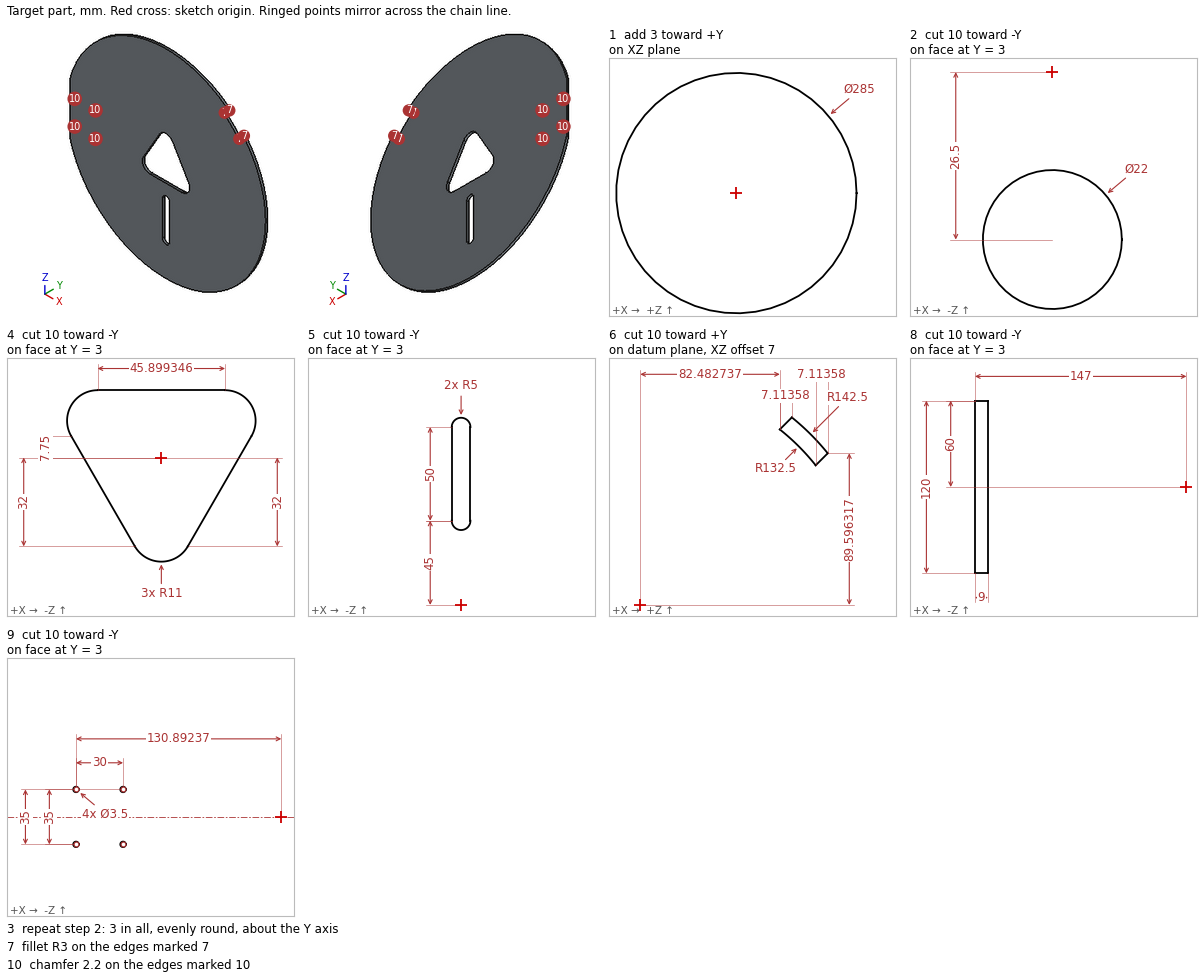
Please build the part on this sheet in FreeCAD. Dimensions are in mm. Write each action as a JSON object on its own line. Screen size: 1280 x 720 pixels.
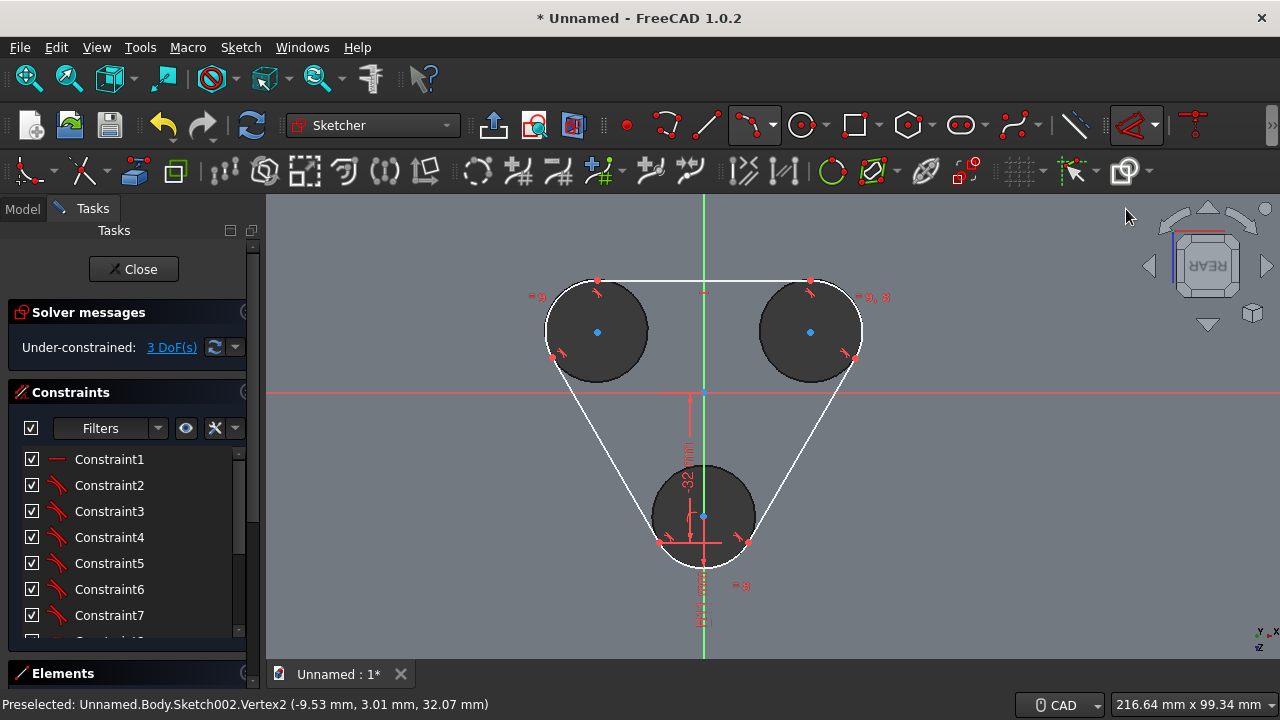
{"action": "left_click", "coordinate": [748, 543]}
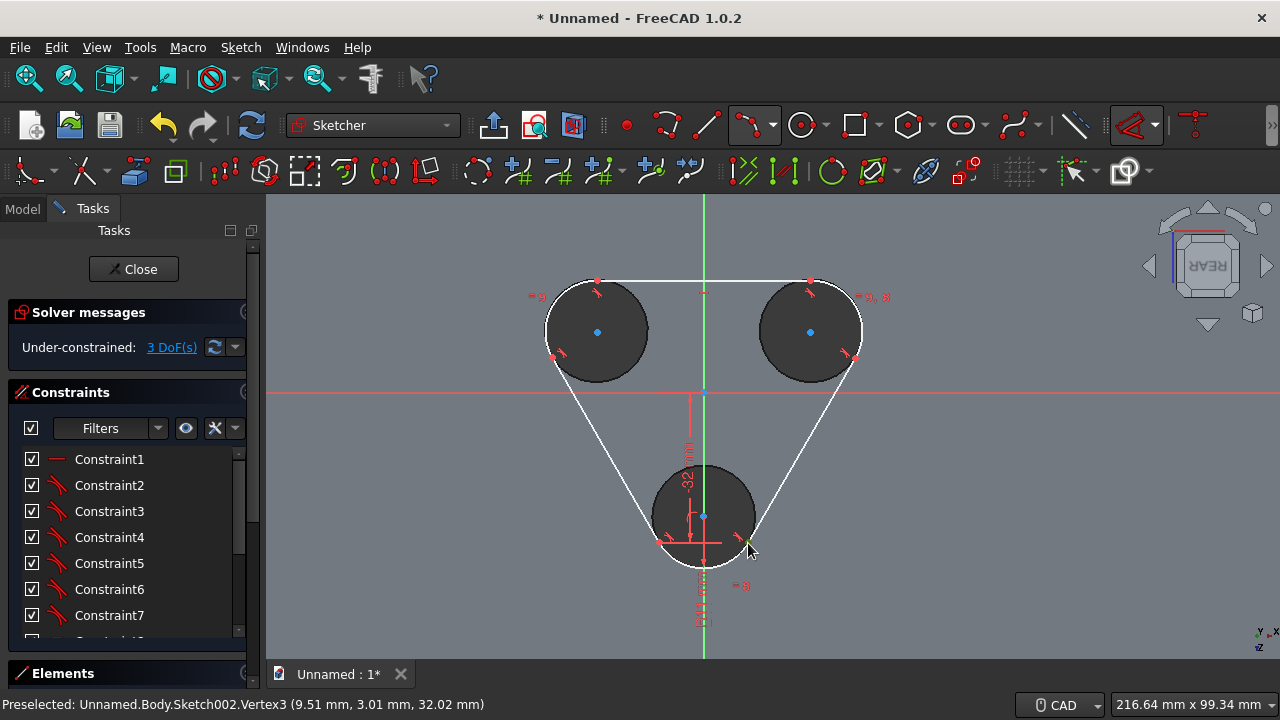
{"action": "key", "text": "i"}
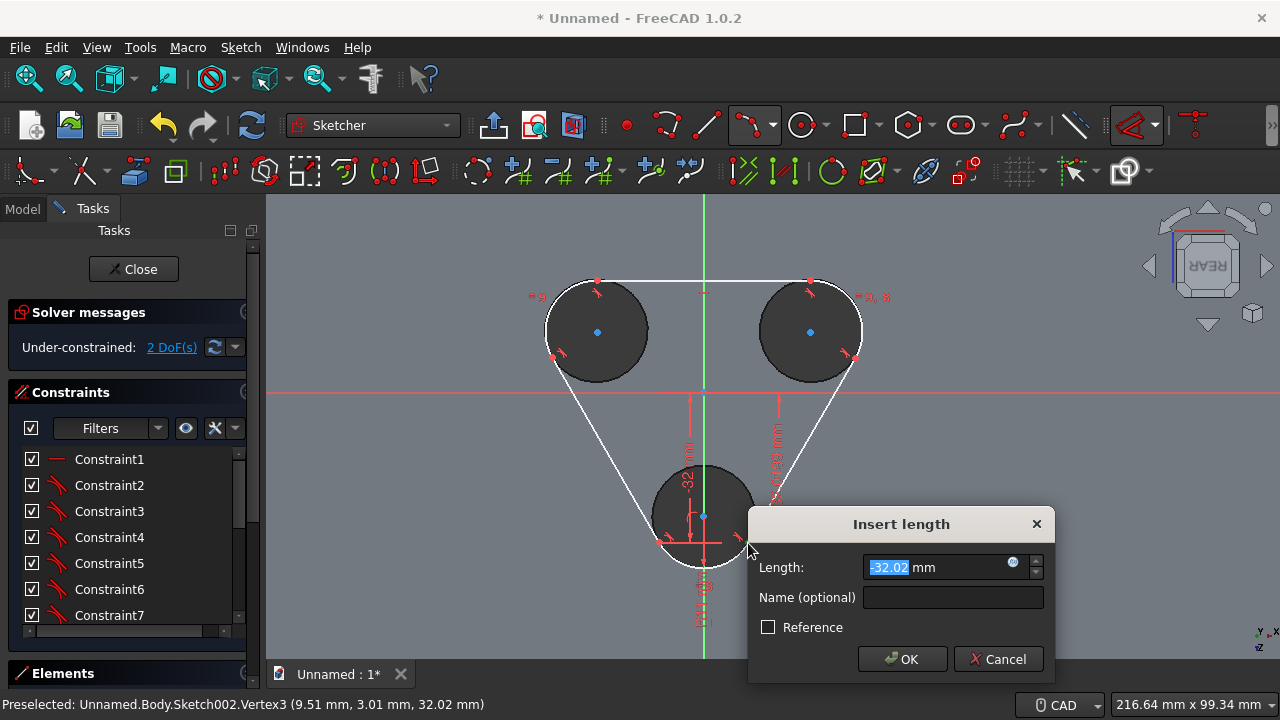
{"action": "type", "text": "-32"}
{"action": "key", "text": "Return"}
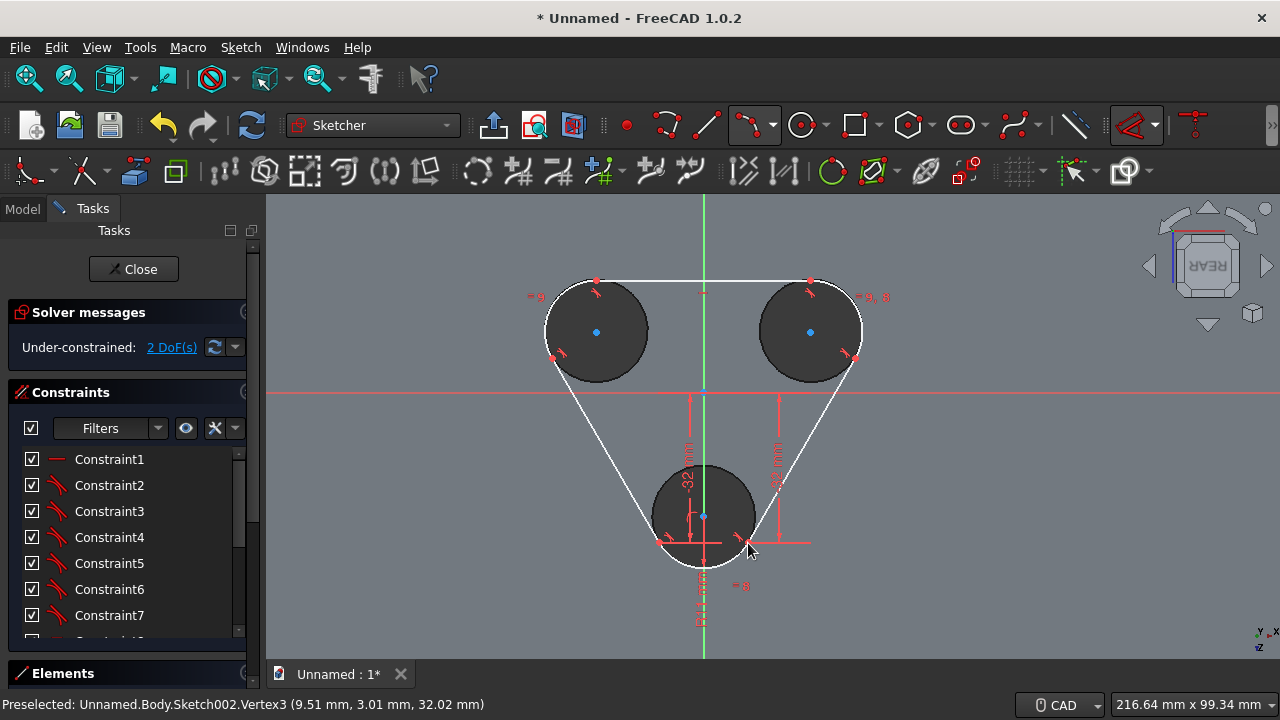
{"action": "left_click", "coordinate": [552, 358]}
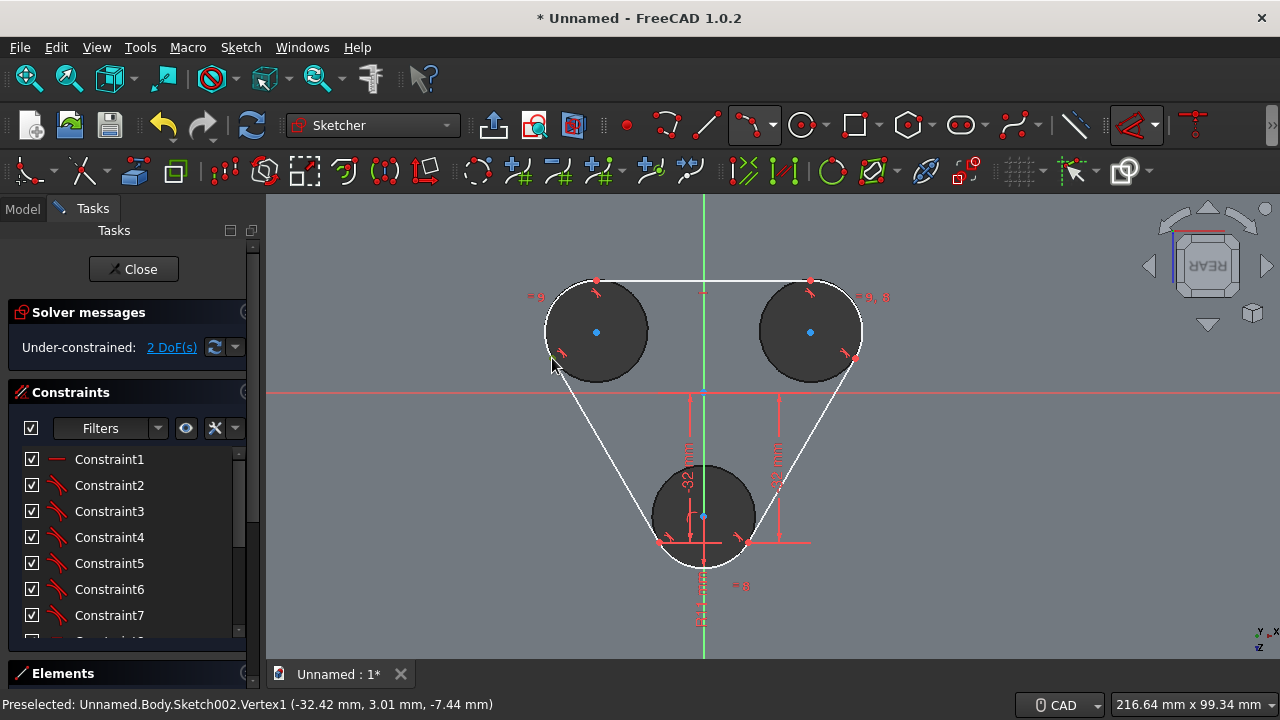
{"action": "left_click", "coordinate": [1158, 126]}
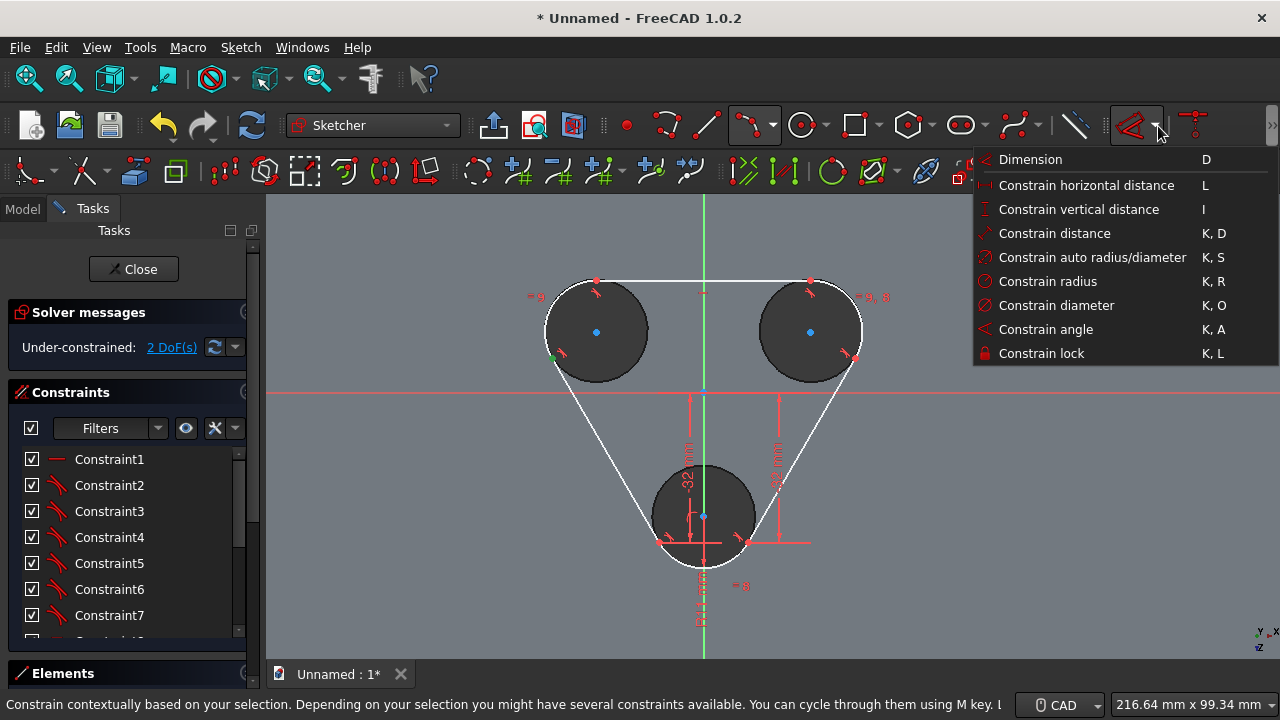
{"action": "left_click", "coordinate": [1126, 209]}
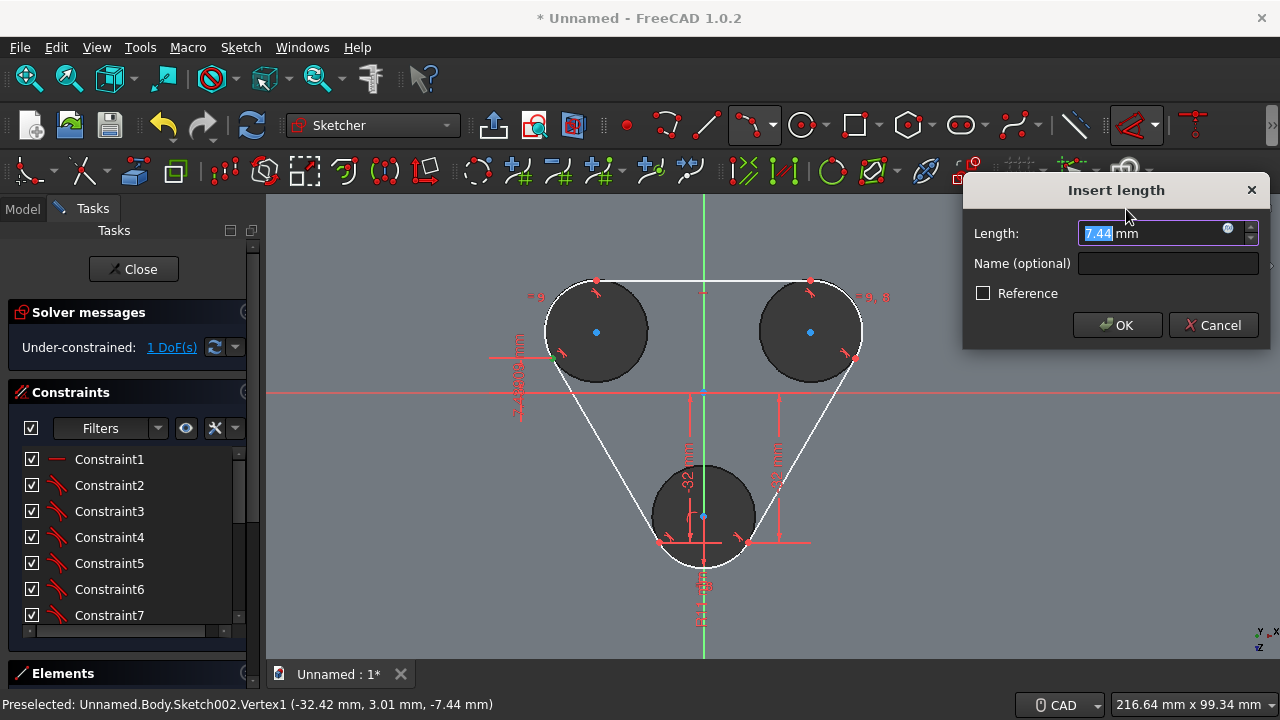
{"action": "type", "text": "7.75"}
{"action": "key", "text": "Return"}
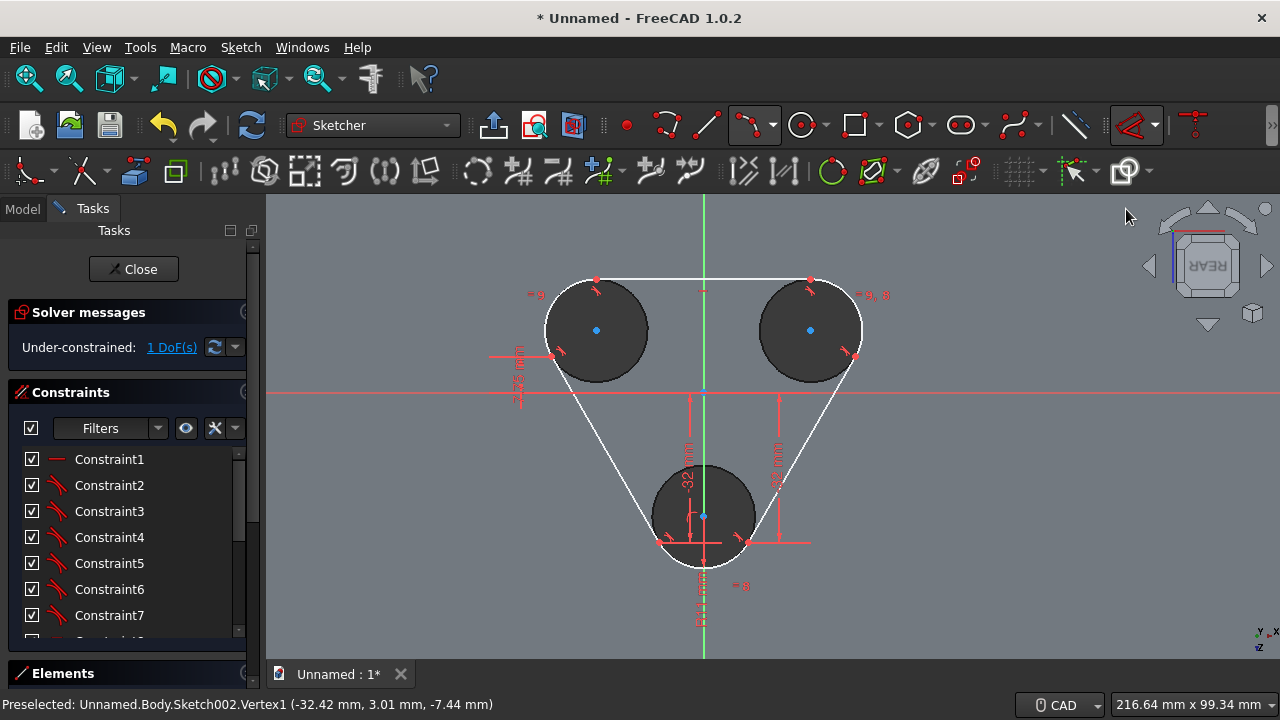
{"action": "left_click", "coordinate": [747, 279]}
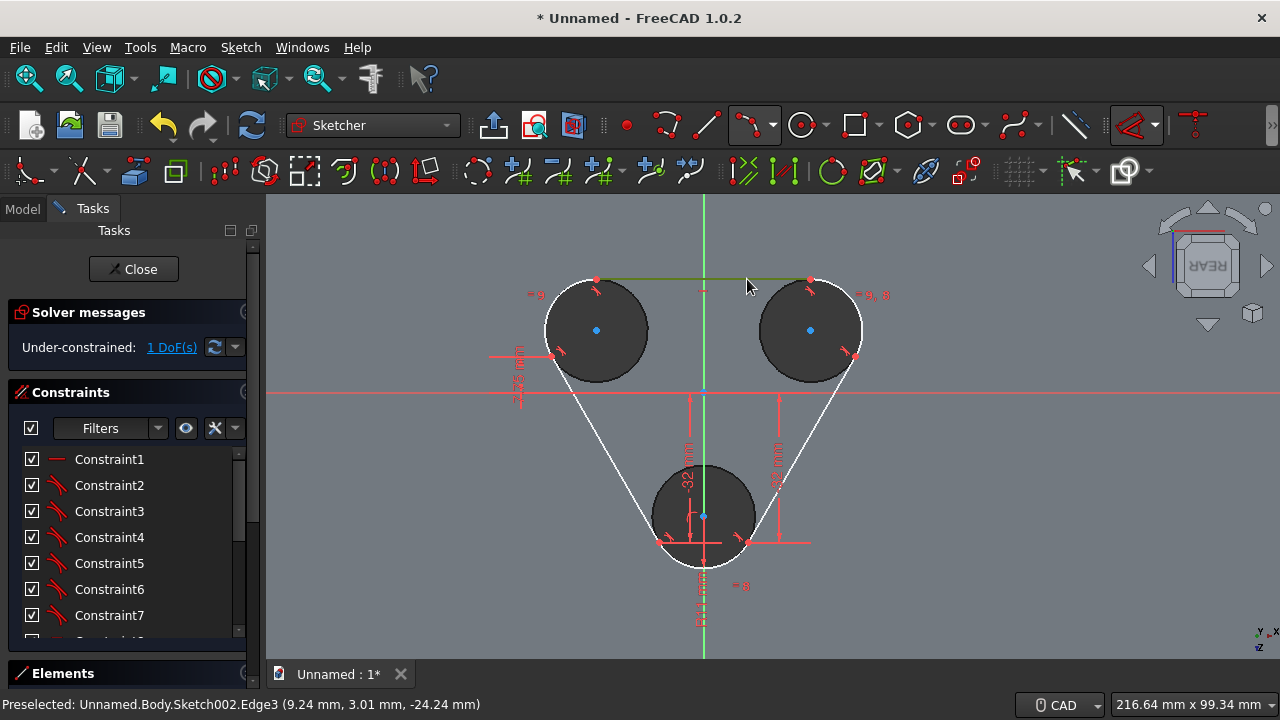
{"action": "left_click", "coordinate": [1158, 126]}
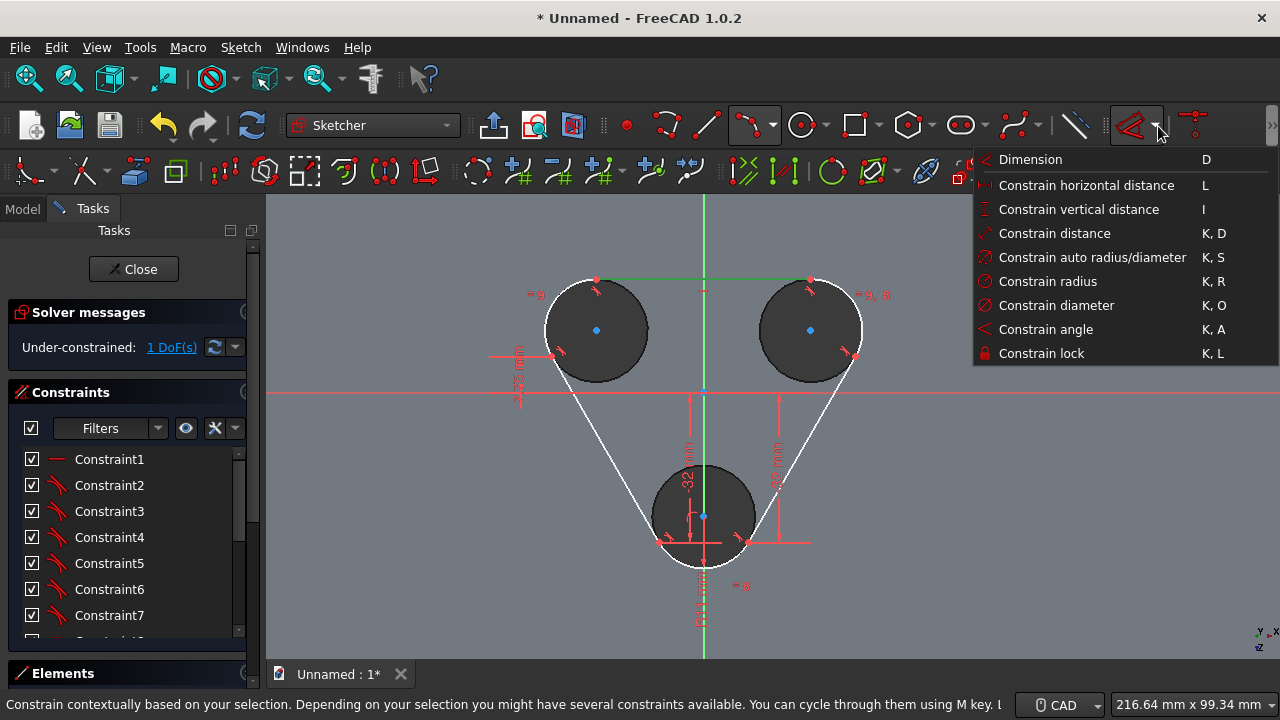
{"action": "left_click", "coordinate": [1126, 185]}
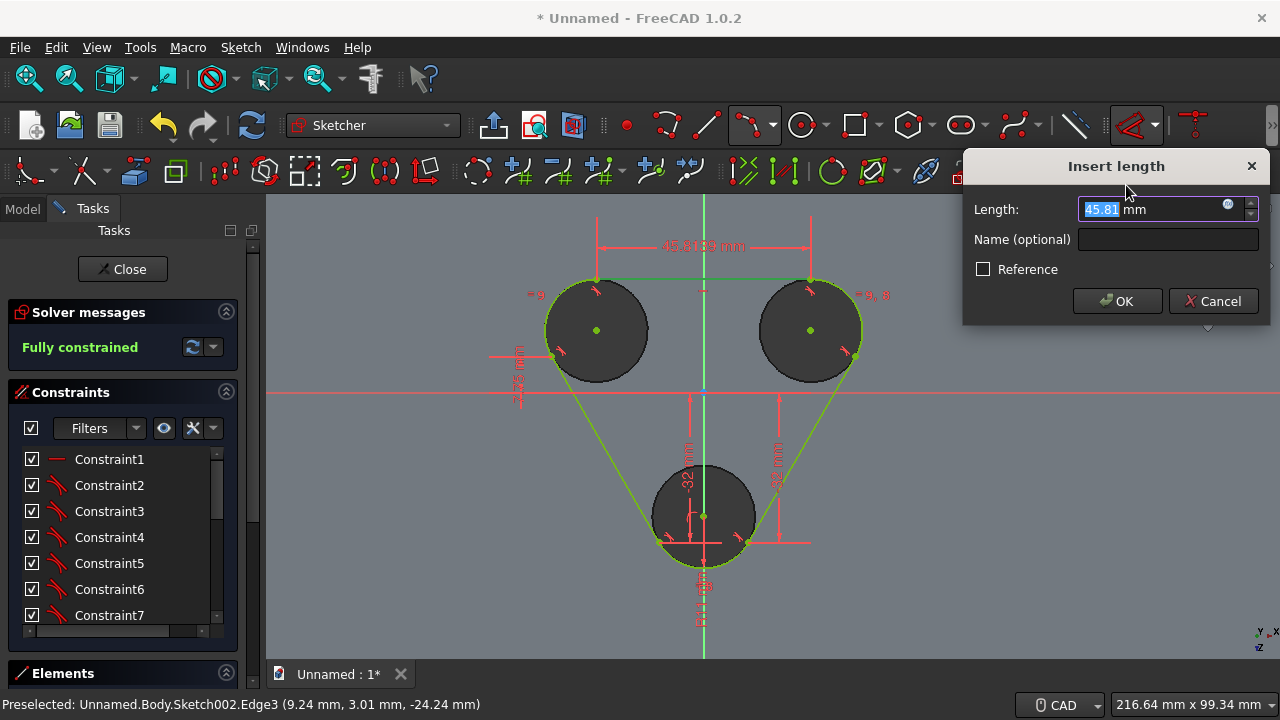
{"action": "type", "text": "45.899346"}
{"action": "key", "text": "Return"}